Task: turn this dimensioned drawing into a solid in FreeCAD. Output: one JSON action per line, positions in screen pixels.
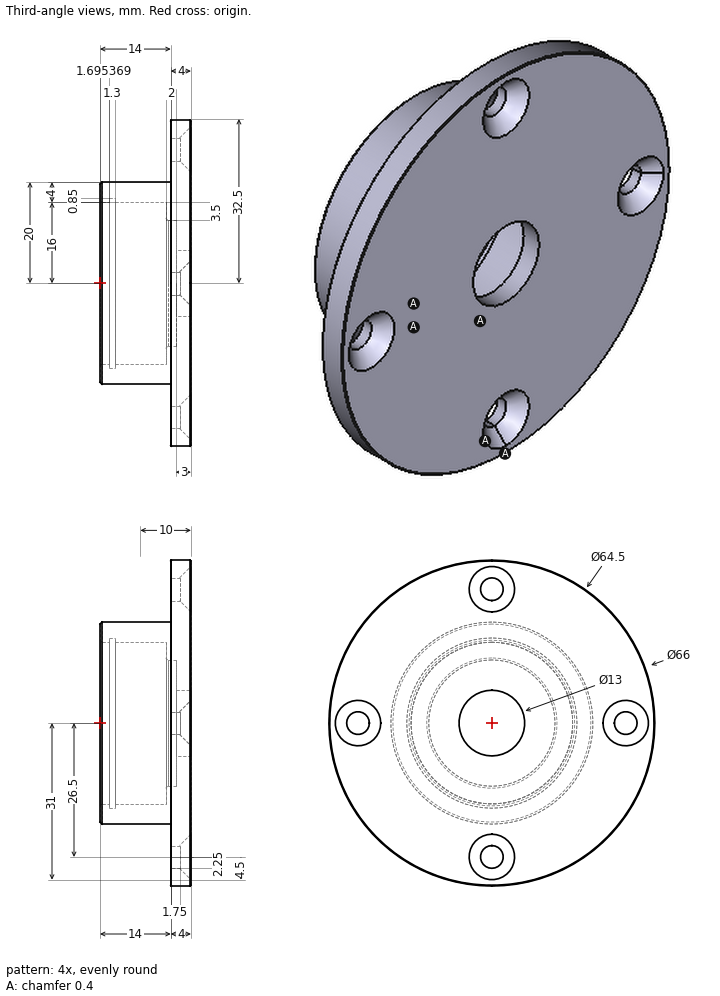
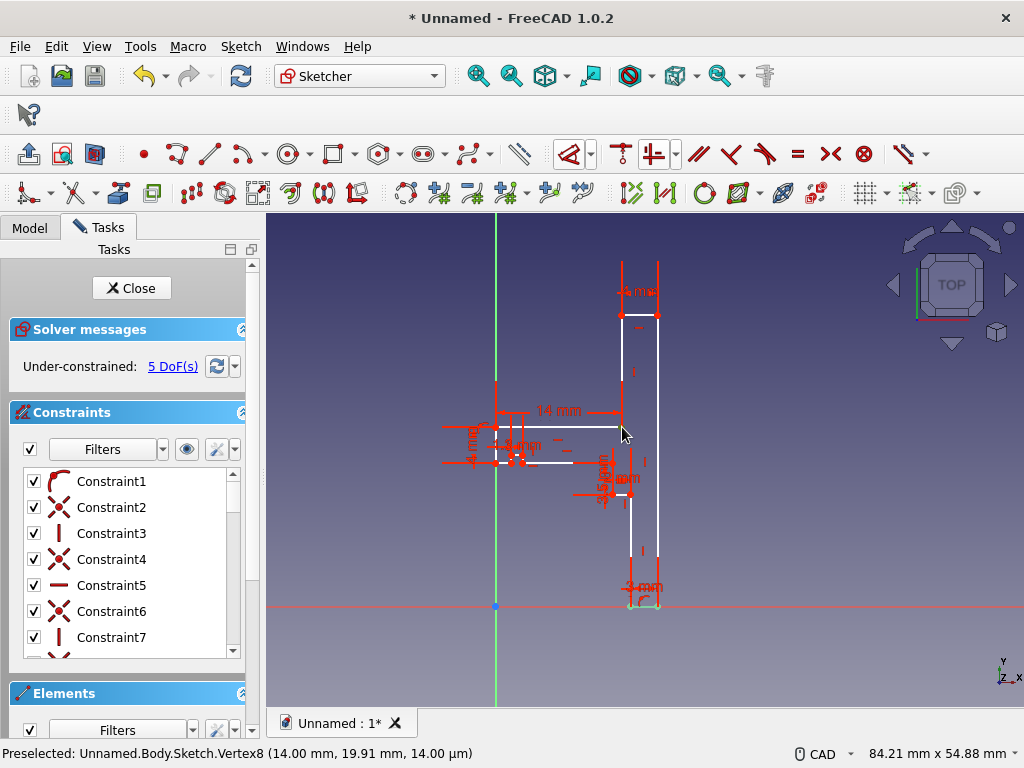
{"action": "left_click", "coordinate": [590, 154]}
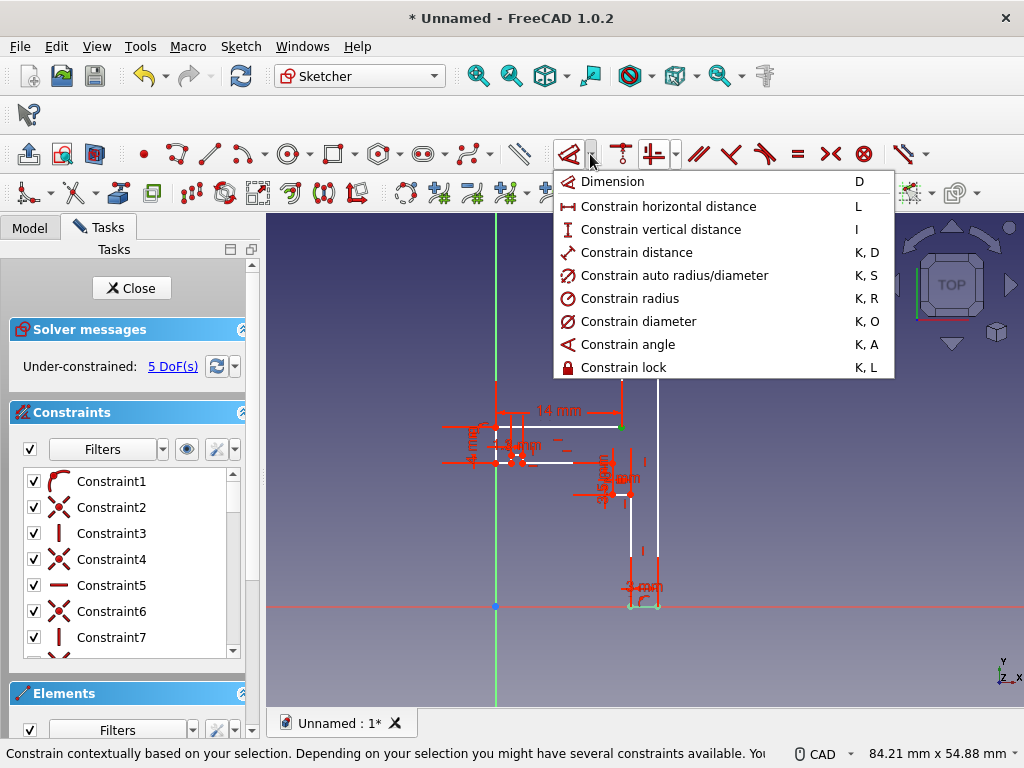
{"action": "left_click", "coordinate": [724, 230]}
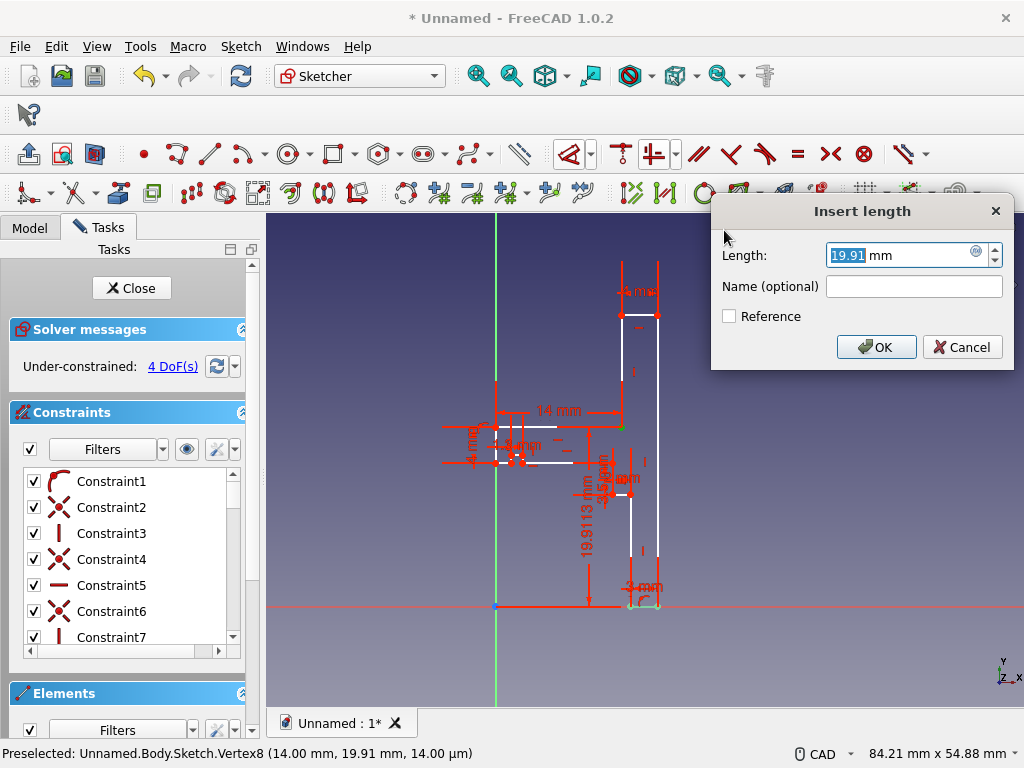
{"action": "type", "text": "20"}
{"action": "key", "text": "Return"}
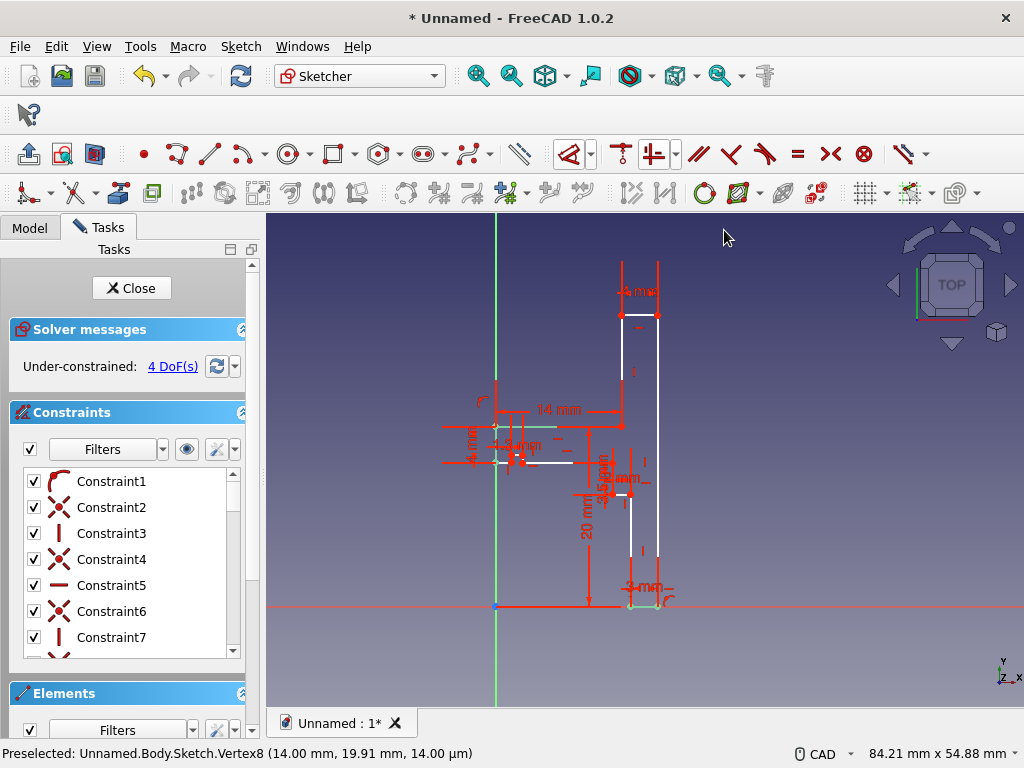
{"action": "scroll", "coordinate": [523, 463], "scroll_direction": "up", "scroll_amount": 3}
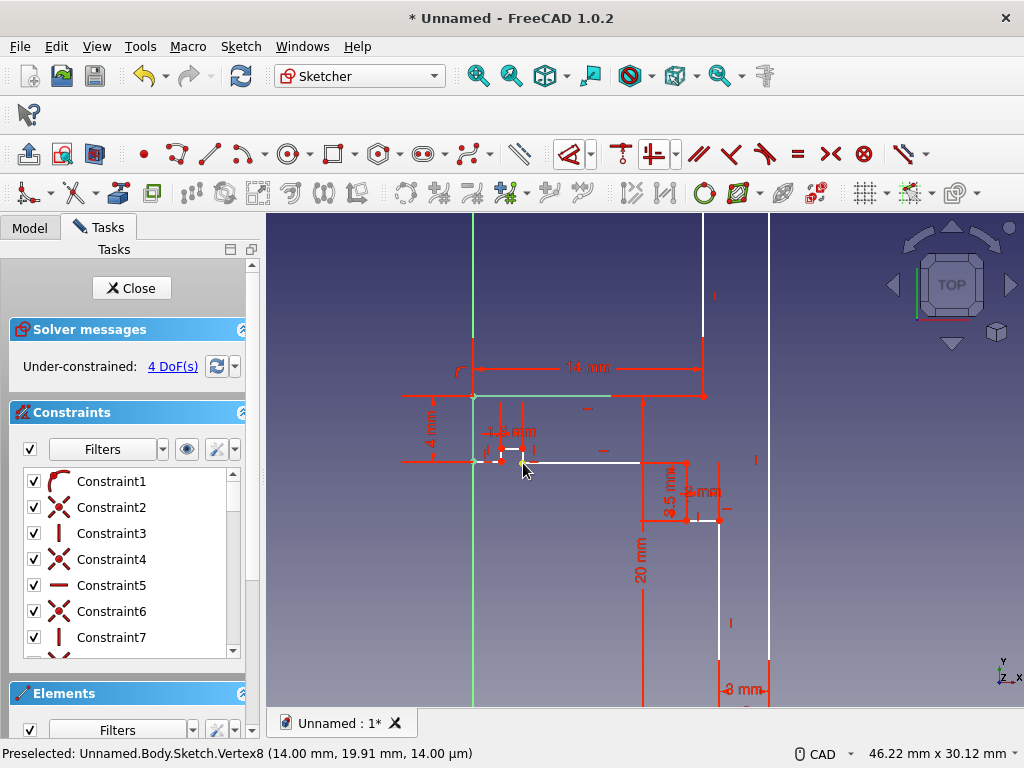
{"action": "left_click", "coordinate": [523, 463]}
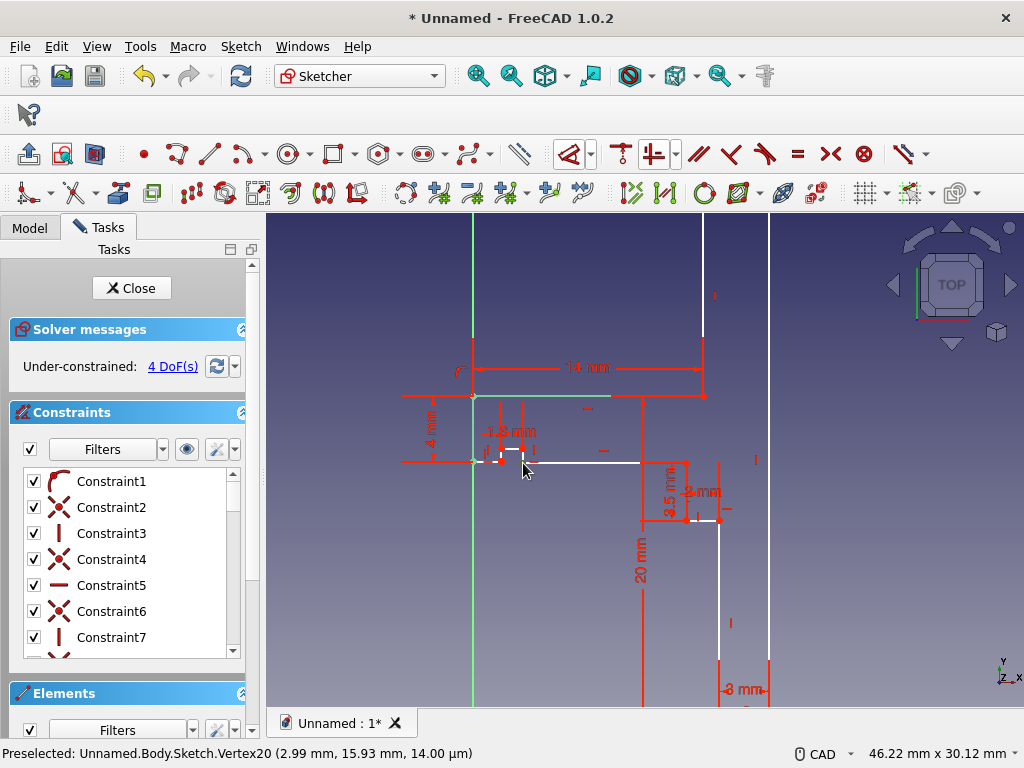
{"action": "key", "text": "i"}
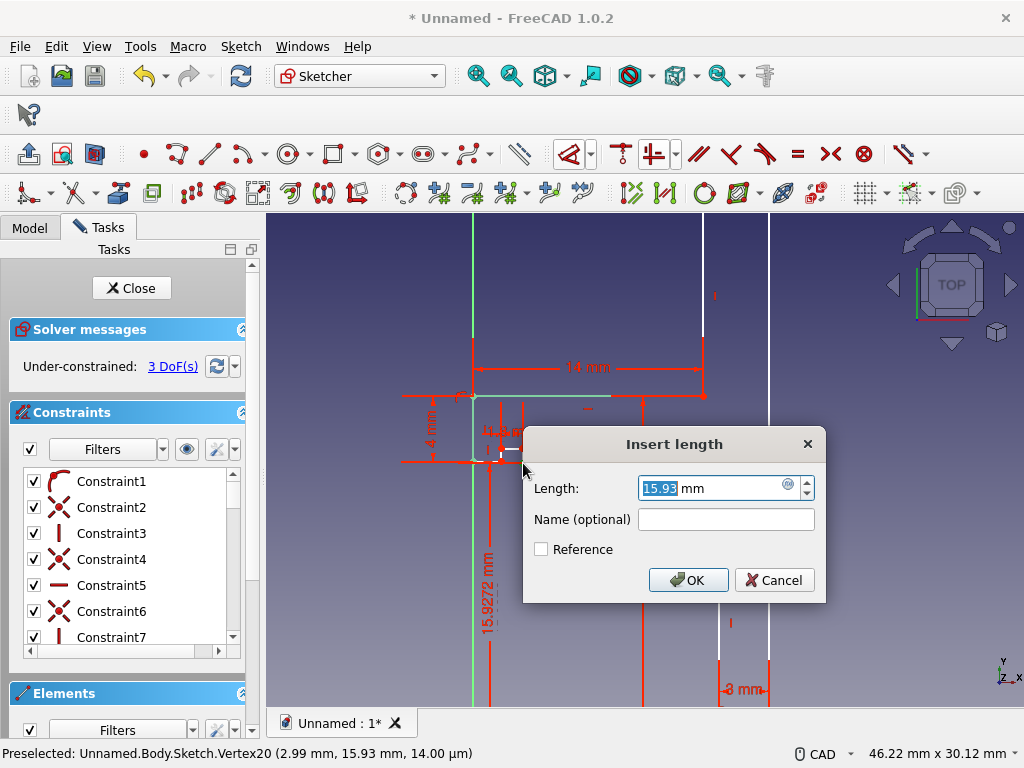
{"action": "type", "text": "16"}
{"action": "key", "text": "Return"}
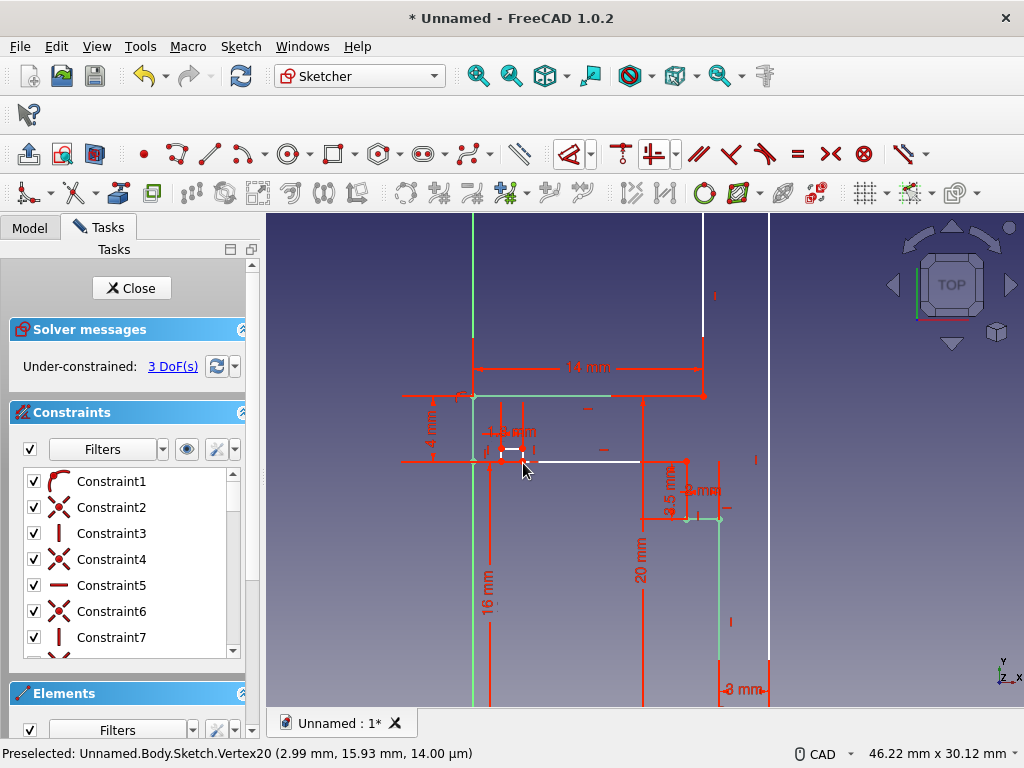
{"action": "left_click", "coordinate": [769, 565]}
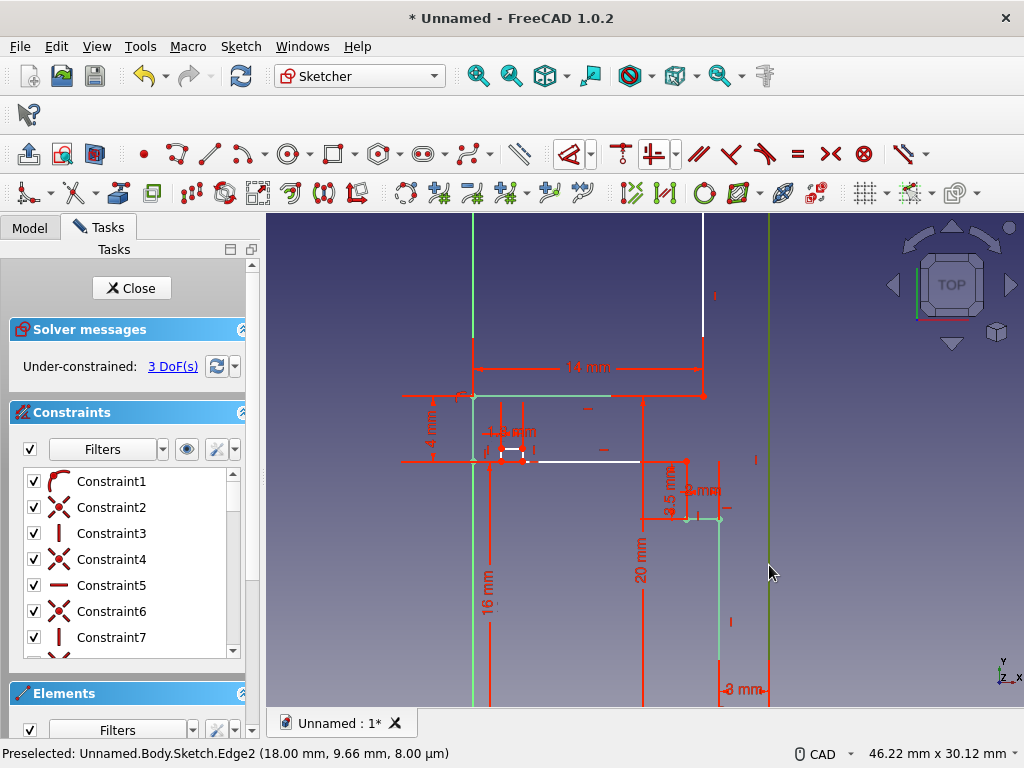
{"action": "key", "text": "i"}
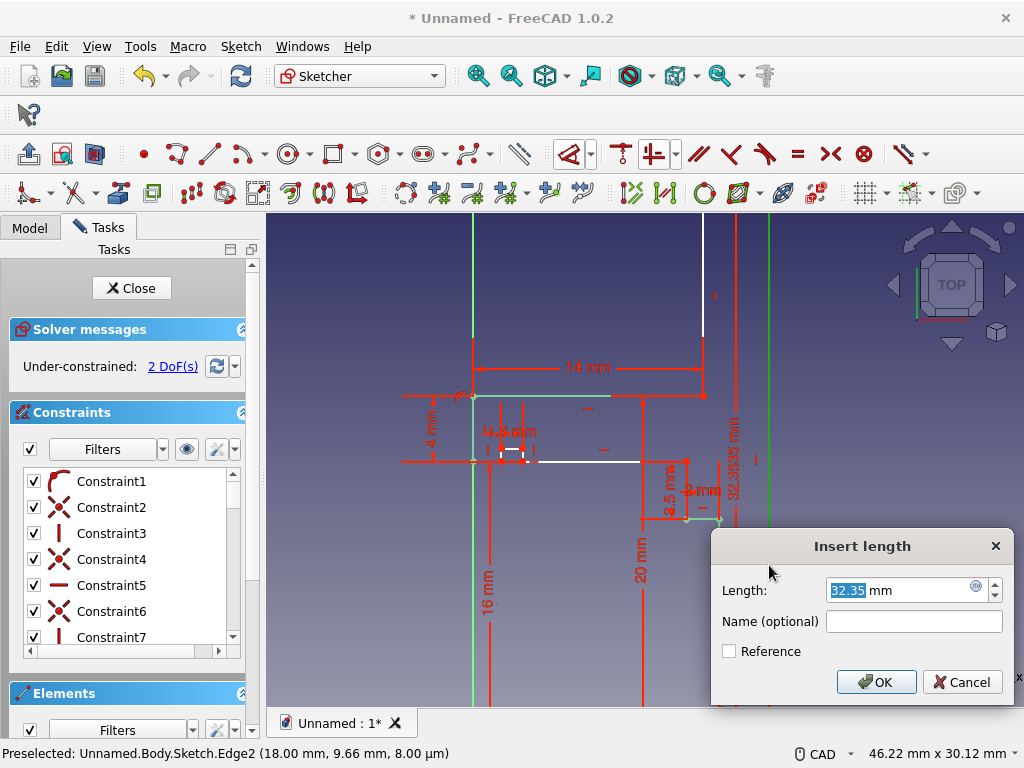
{"action": "type", "text": "32.5"}
{"action": "key", "text": "Return"}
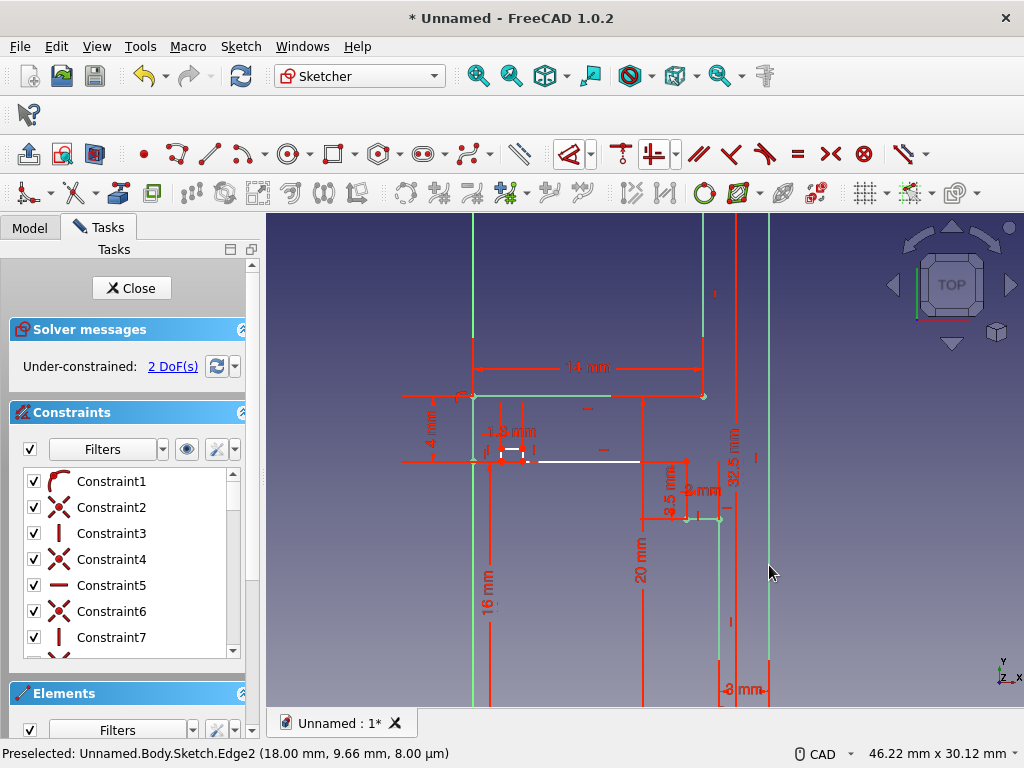
{"action": "scroll", "coordinate": [501, 455], "scroll_direction": "up", "scroll_amount": 6}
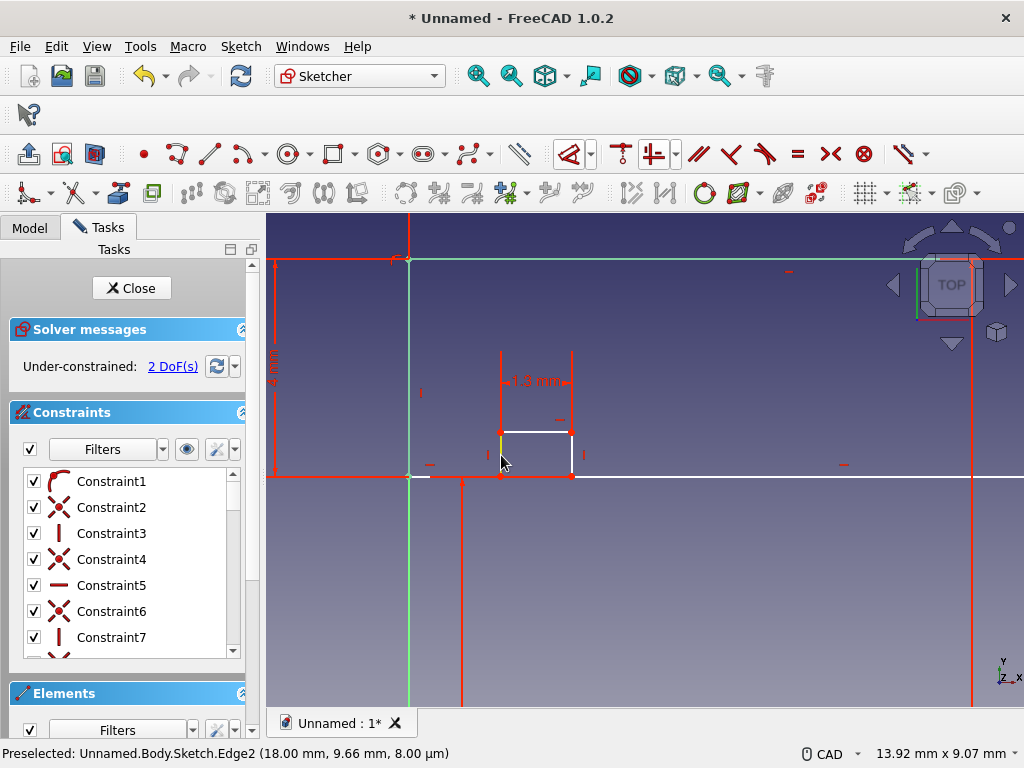
{"action": "left_click", "coordinate": [501, 455]}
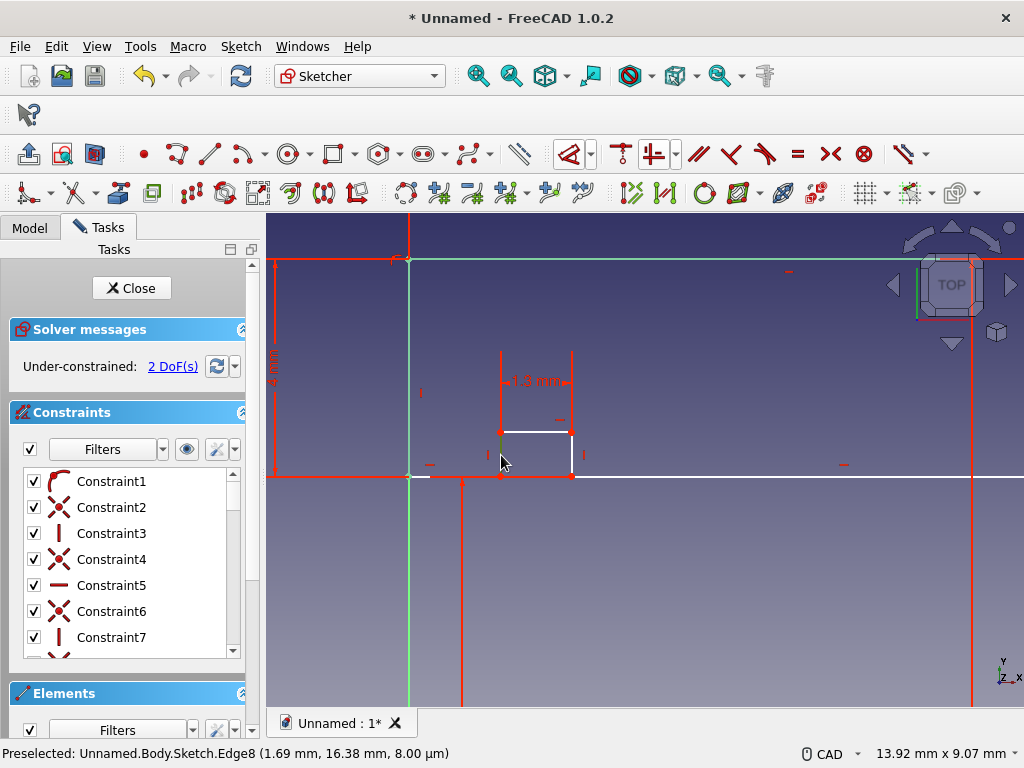
{"action": "left_click", "coordinate": [590, 154]}